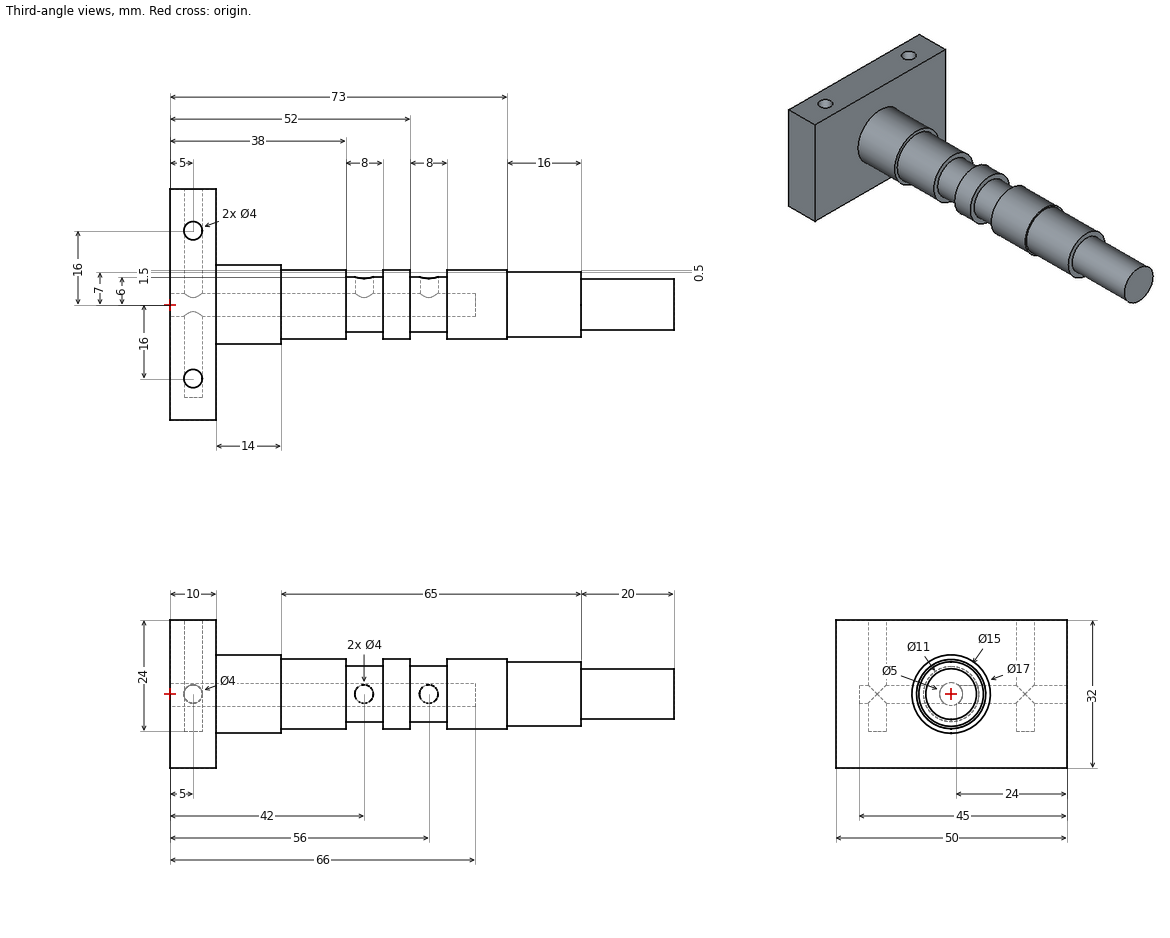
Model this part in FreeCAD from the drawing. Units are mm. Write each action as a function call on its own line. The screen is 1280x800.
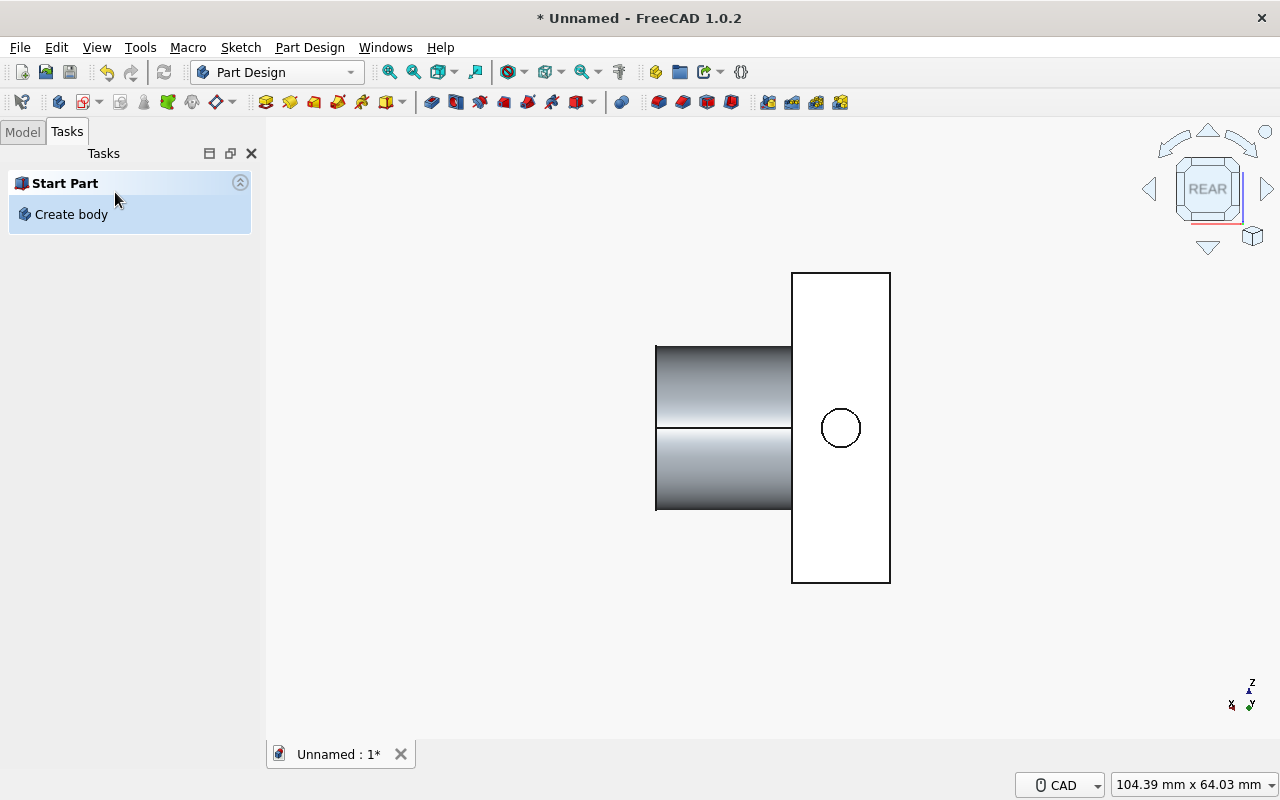
key(0)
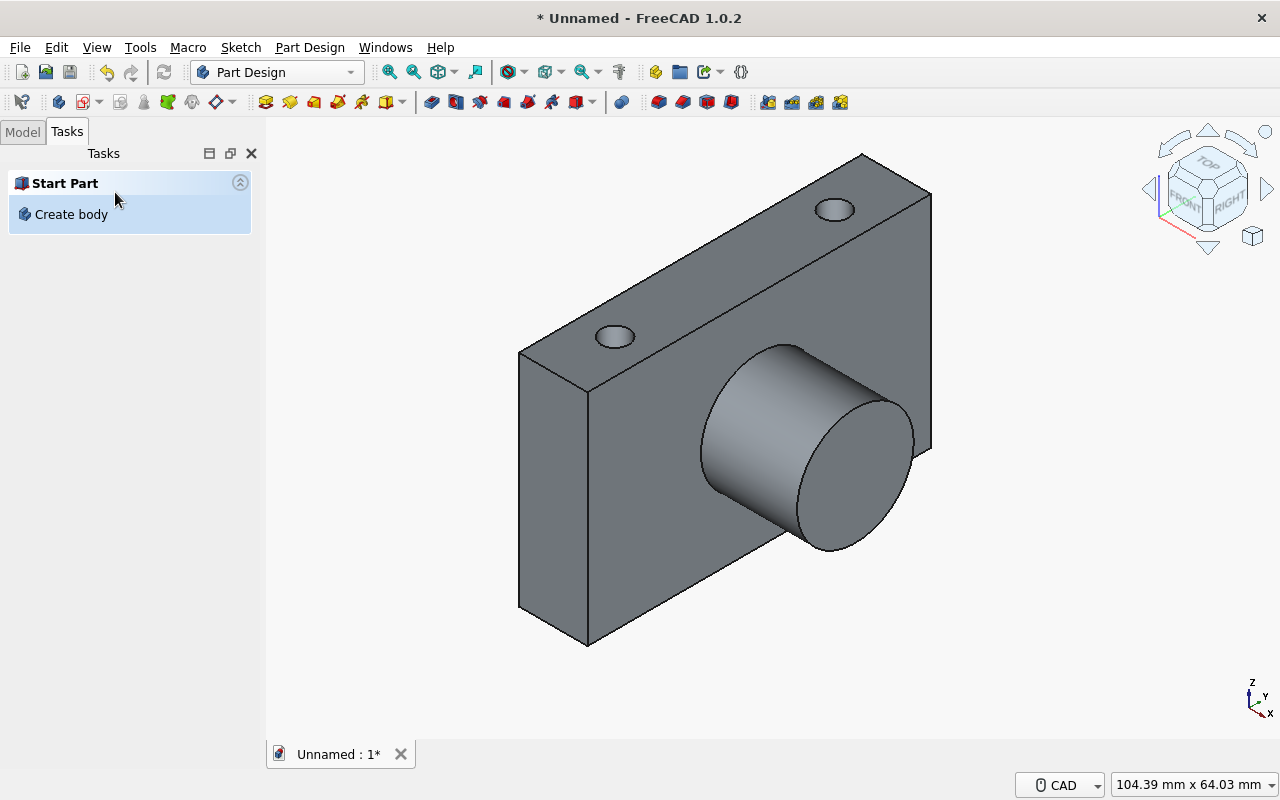
click(855, 475)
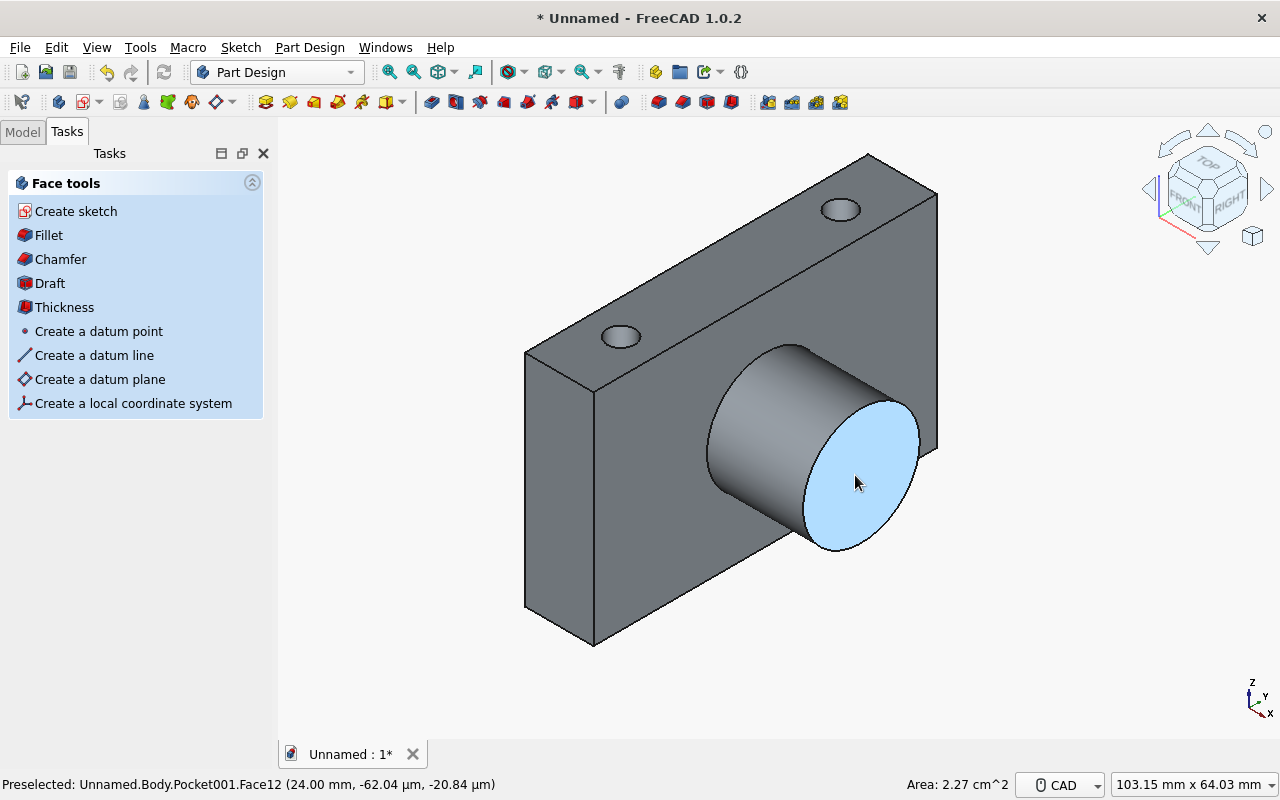
click(84, 102)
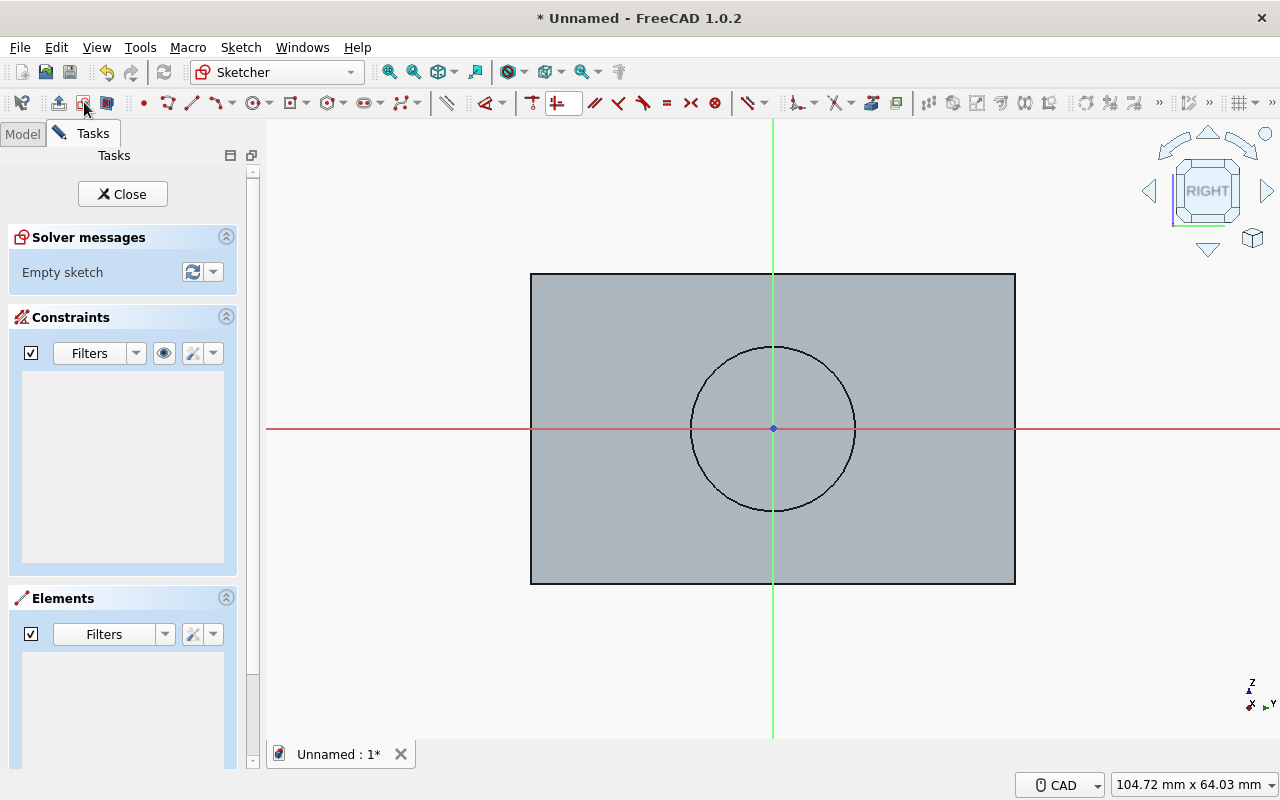
scroll(813, 429, up, 5)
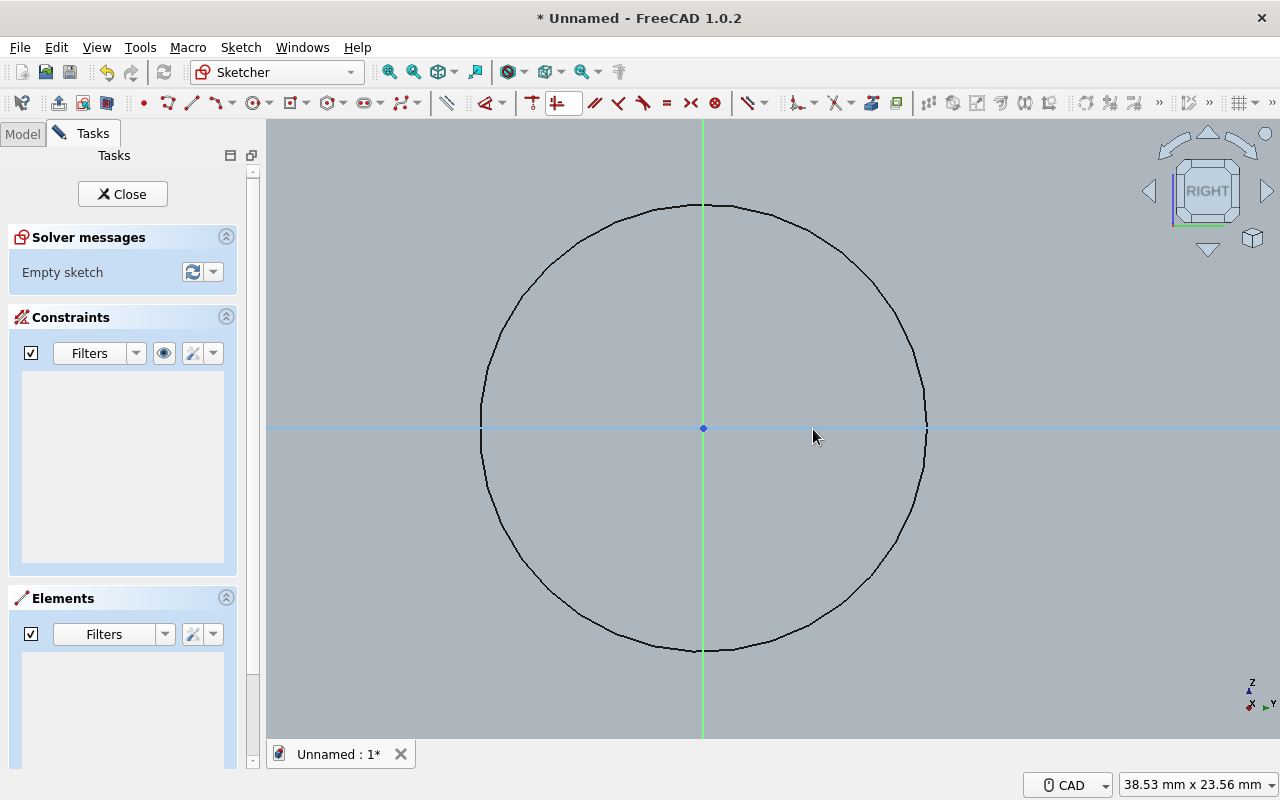
click(254, 104)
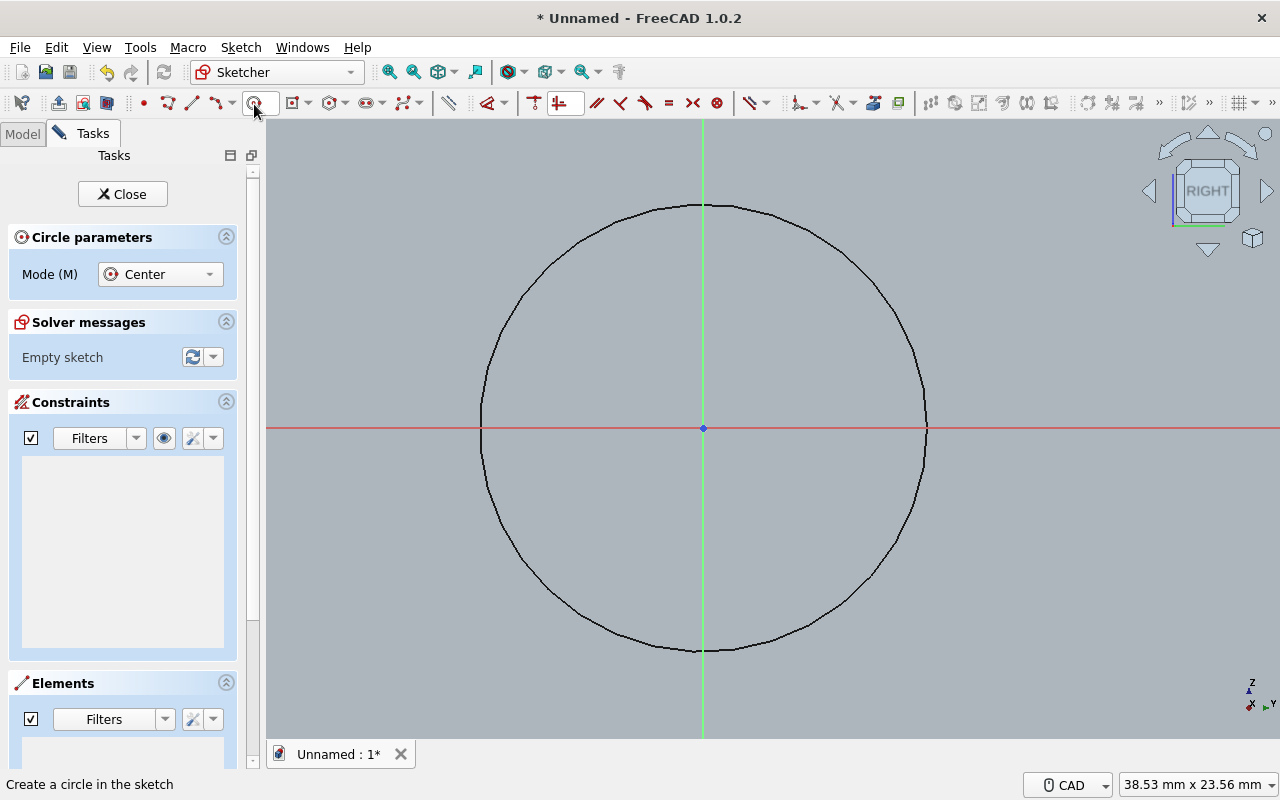
click(703, 428)
move(843, 289)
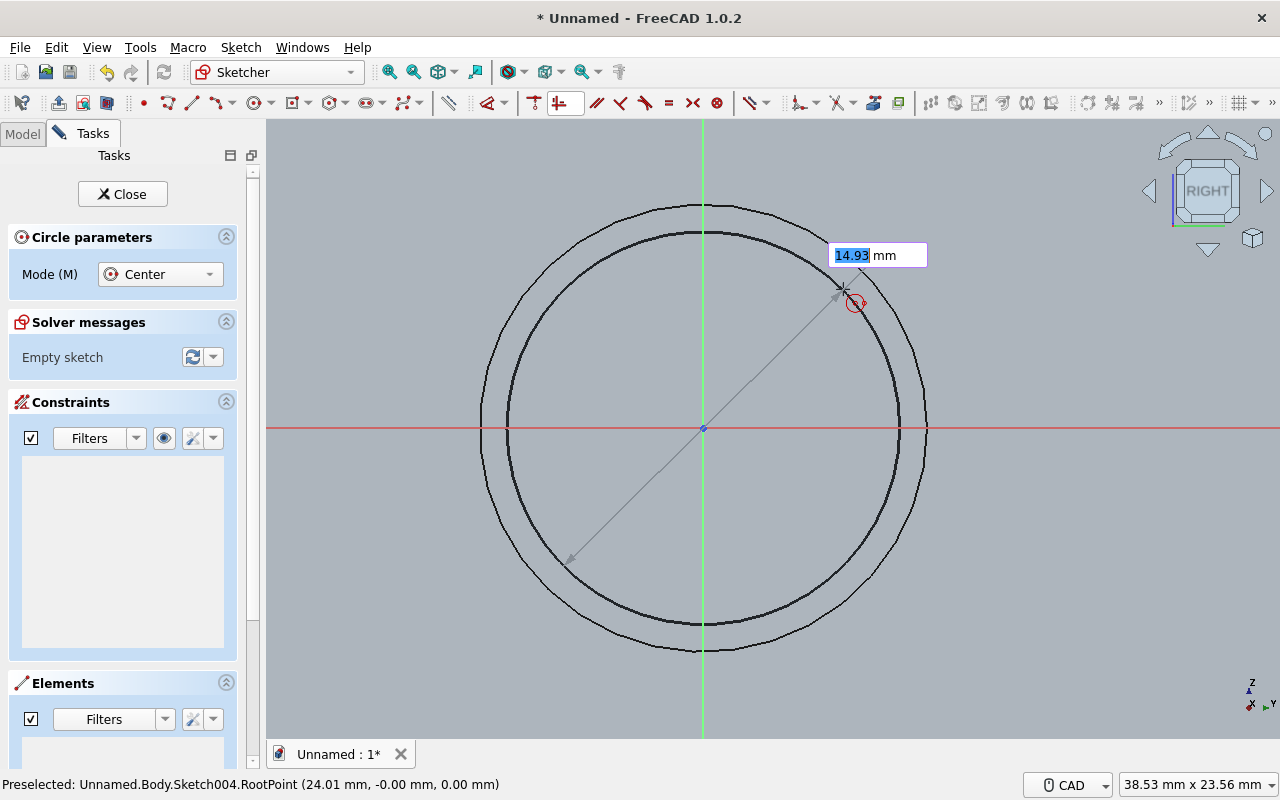
text(15)
key(Return)
key(Escape)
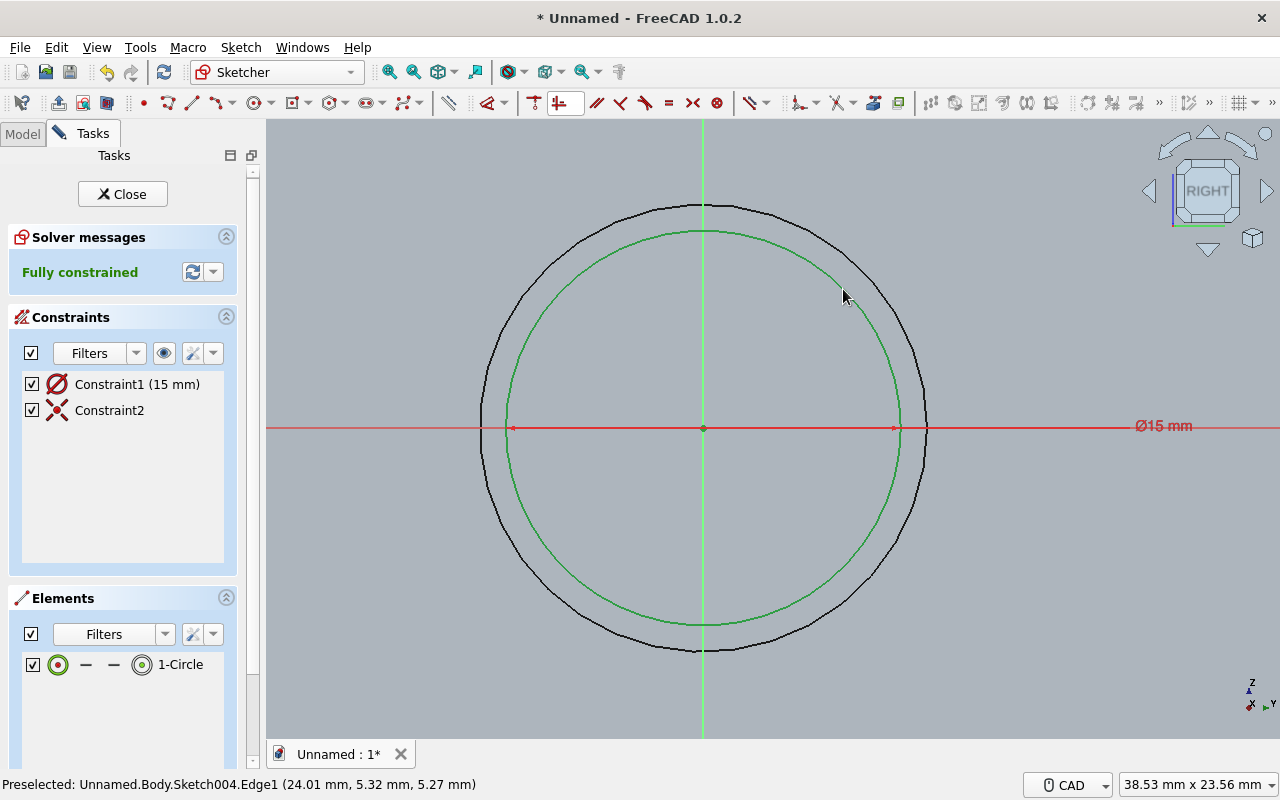
click(123, 194)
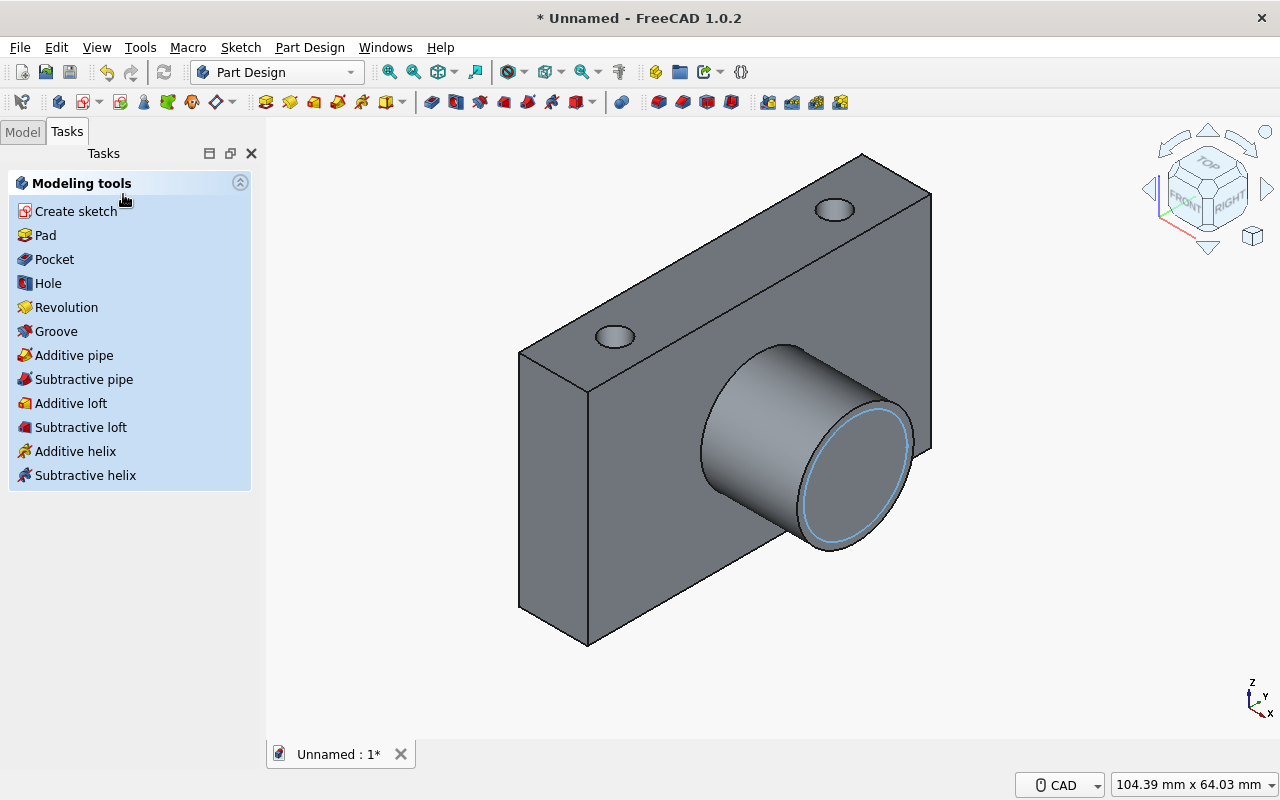
click(266, 102)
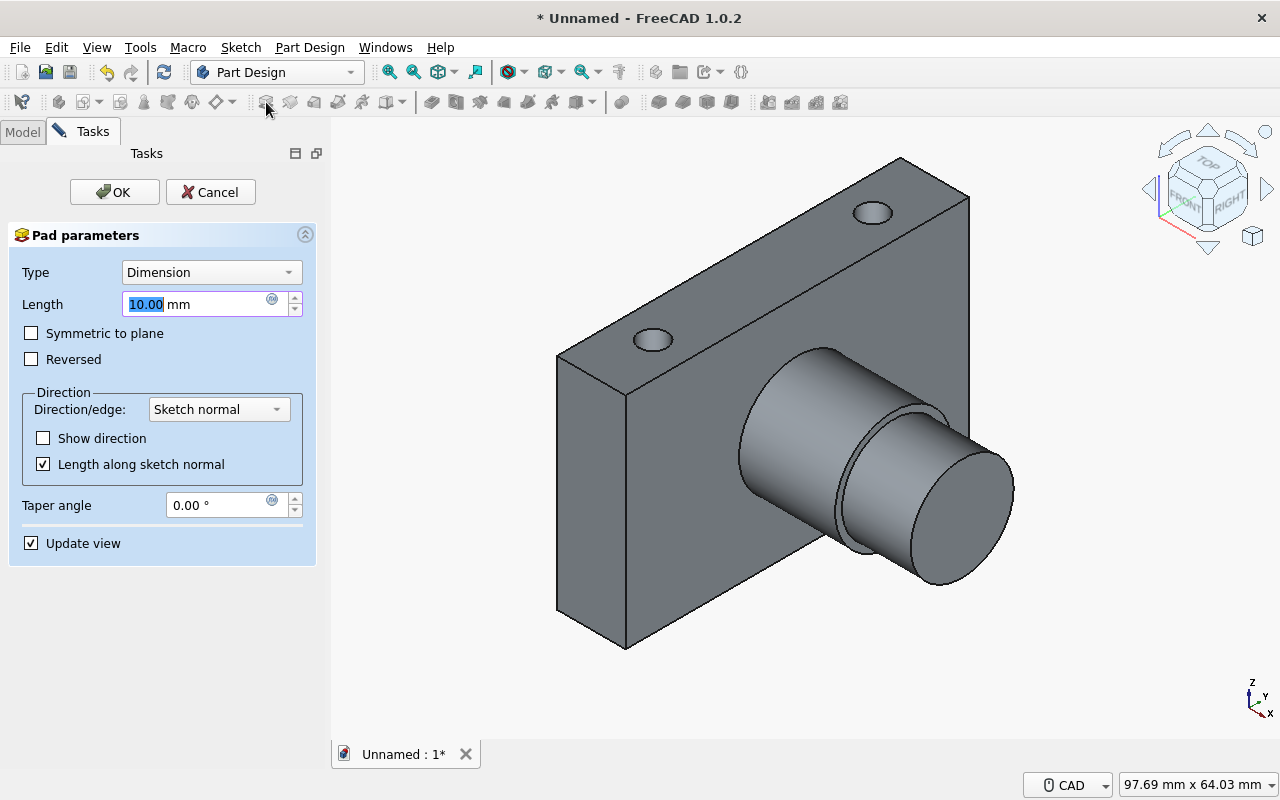
text(65)
key(Tab)